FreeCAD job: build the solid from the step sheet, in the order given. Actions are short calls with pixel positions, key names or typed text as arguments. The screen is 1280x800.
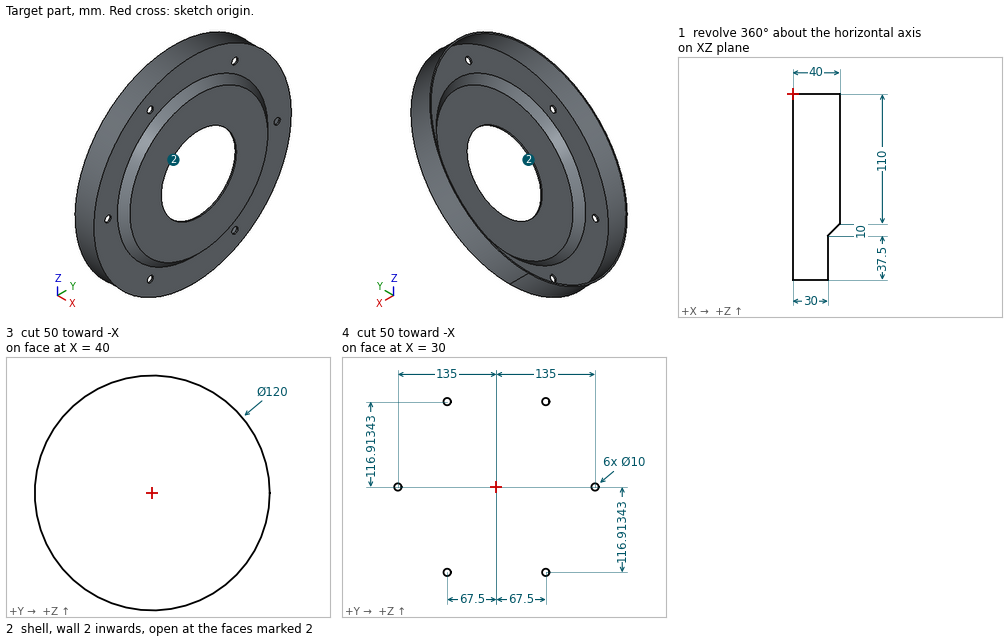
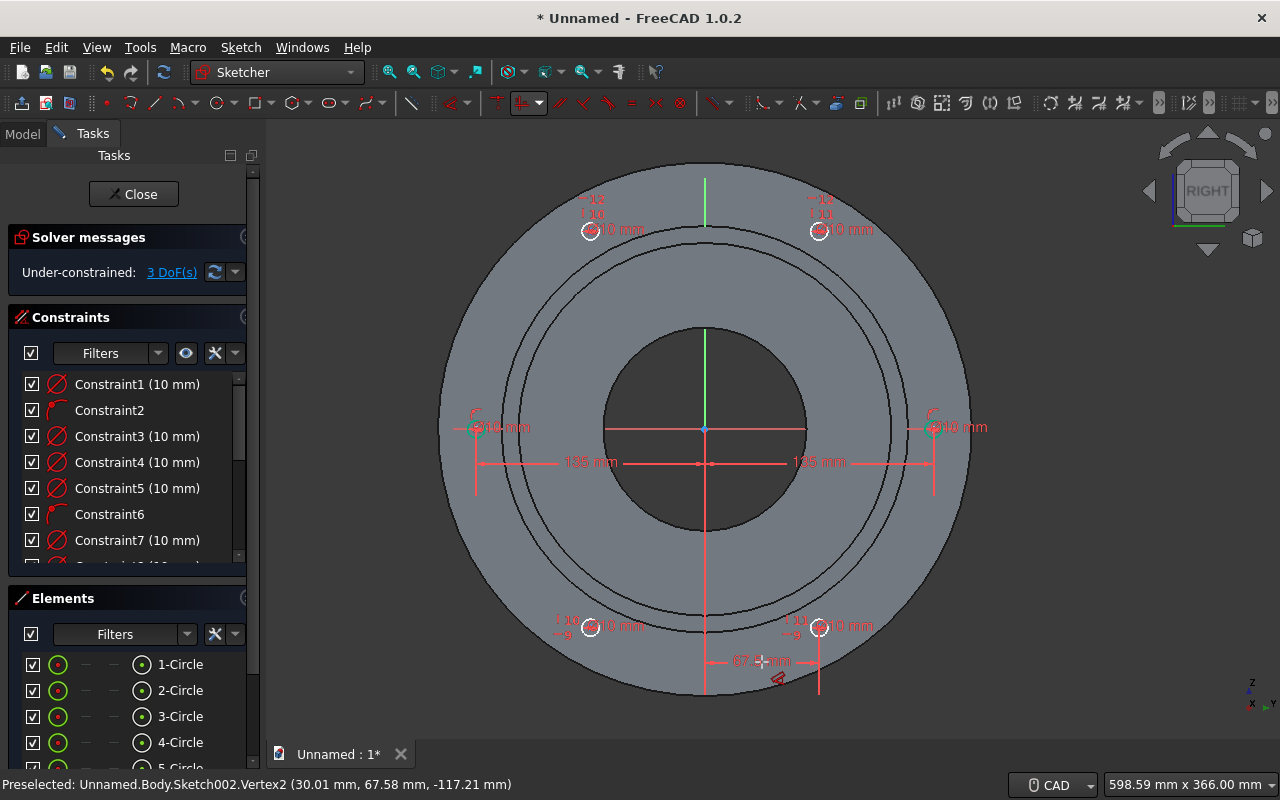
click(590, 628)
click(648, 662)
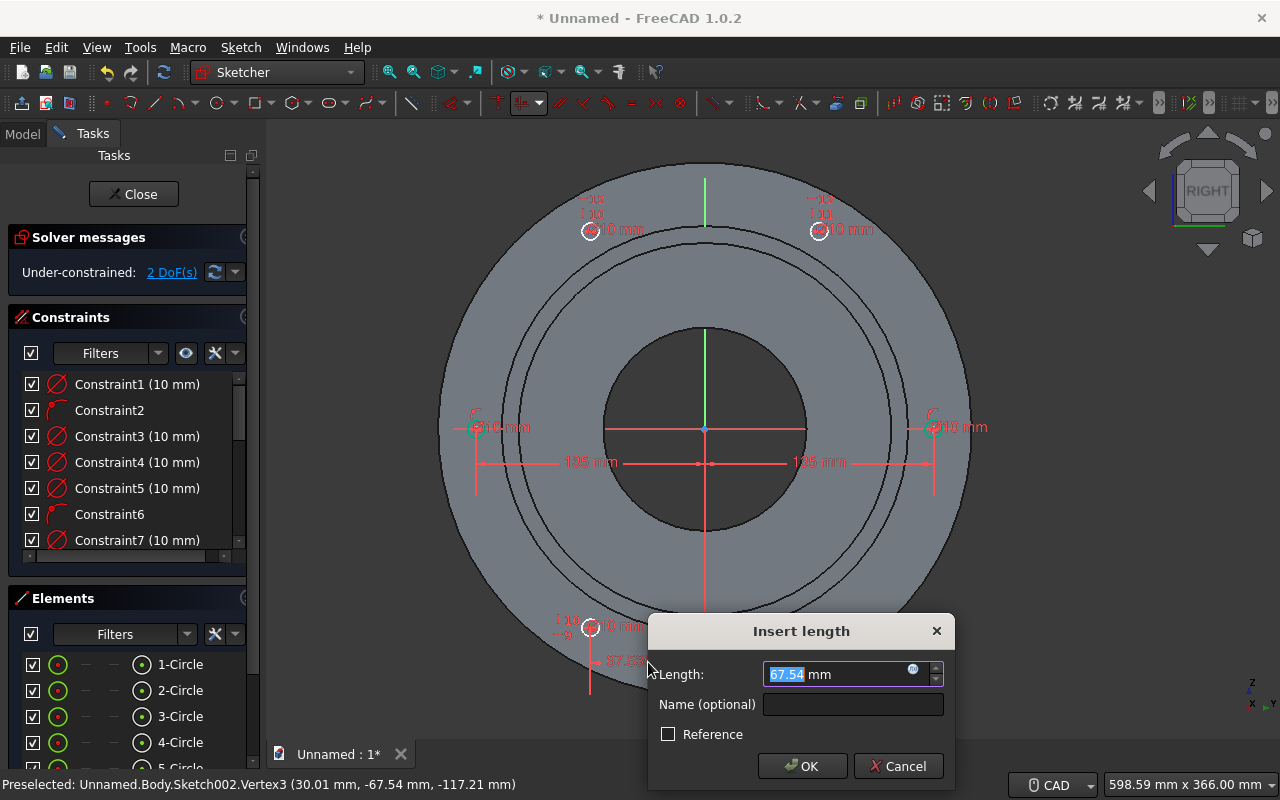
text(67.5)
key(Return)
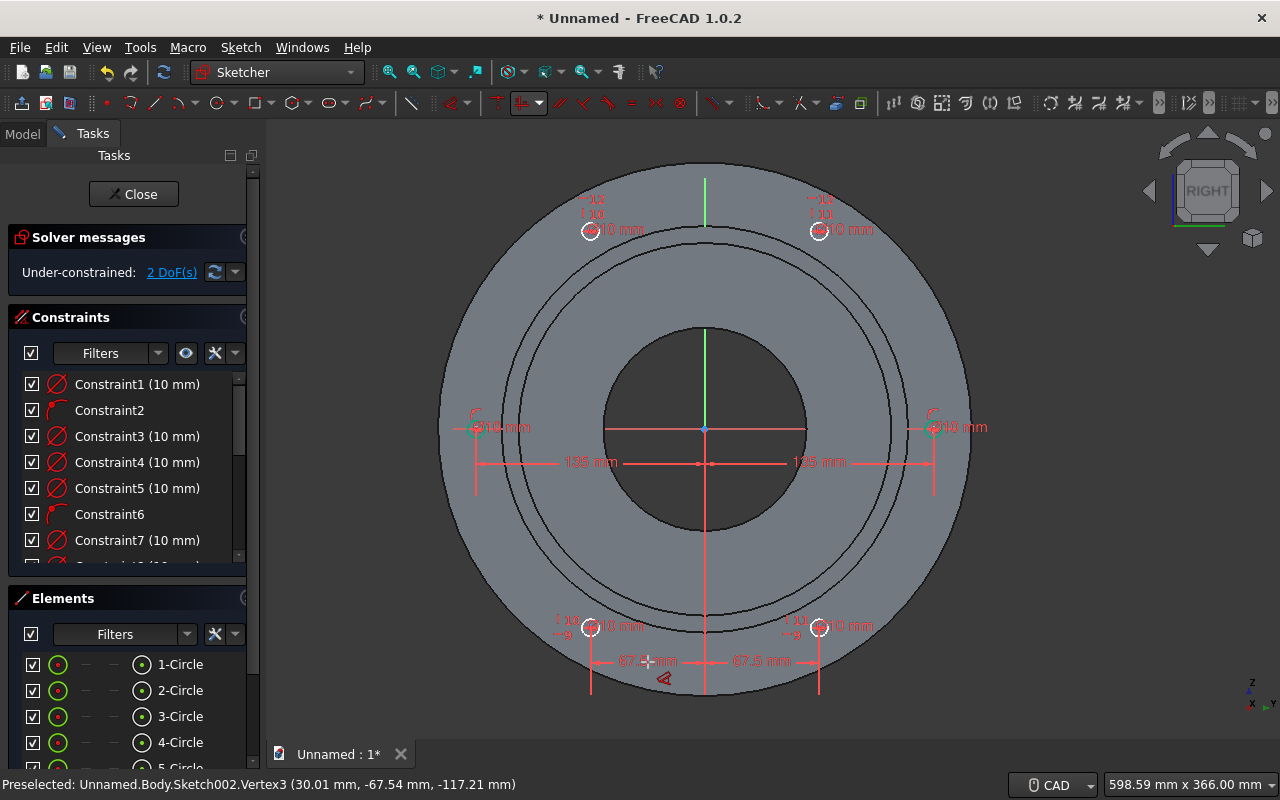
click(819, 628)
click(853, 529)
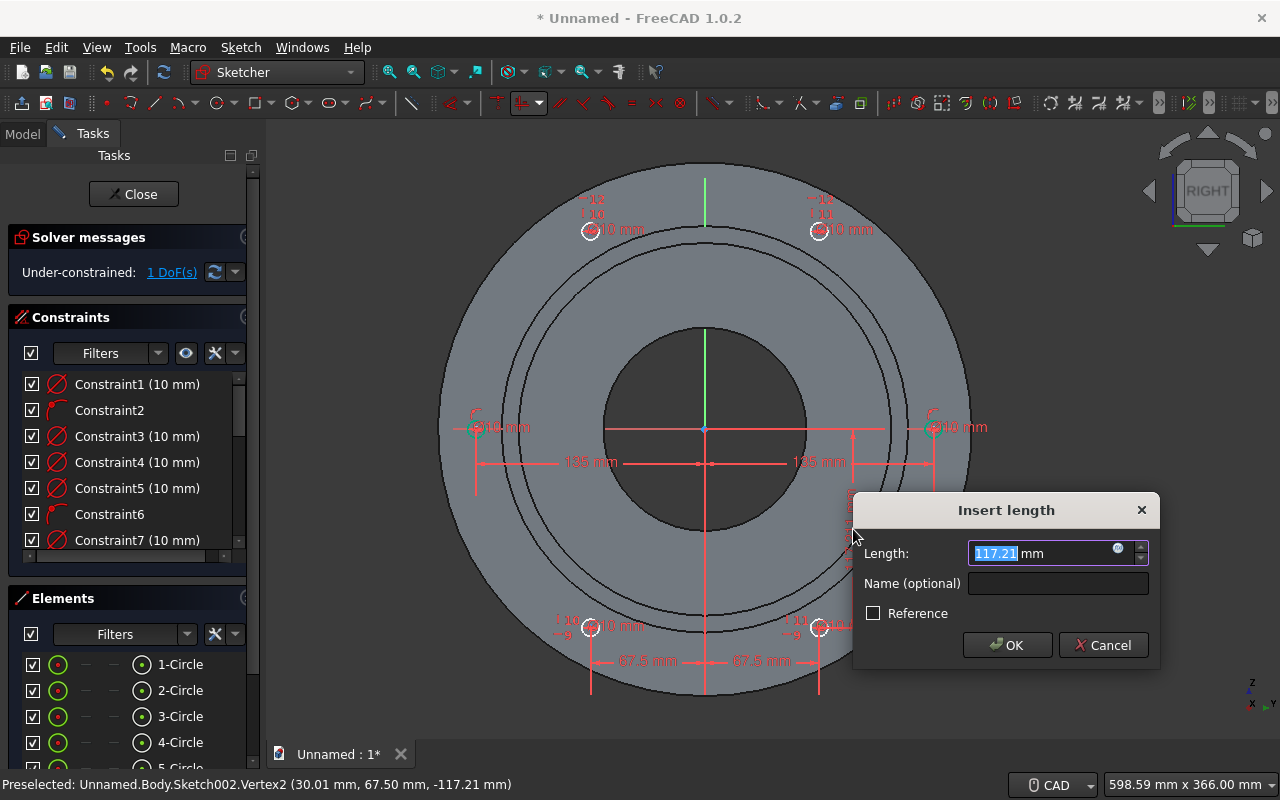
text(116.91343)
key(Return)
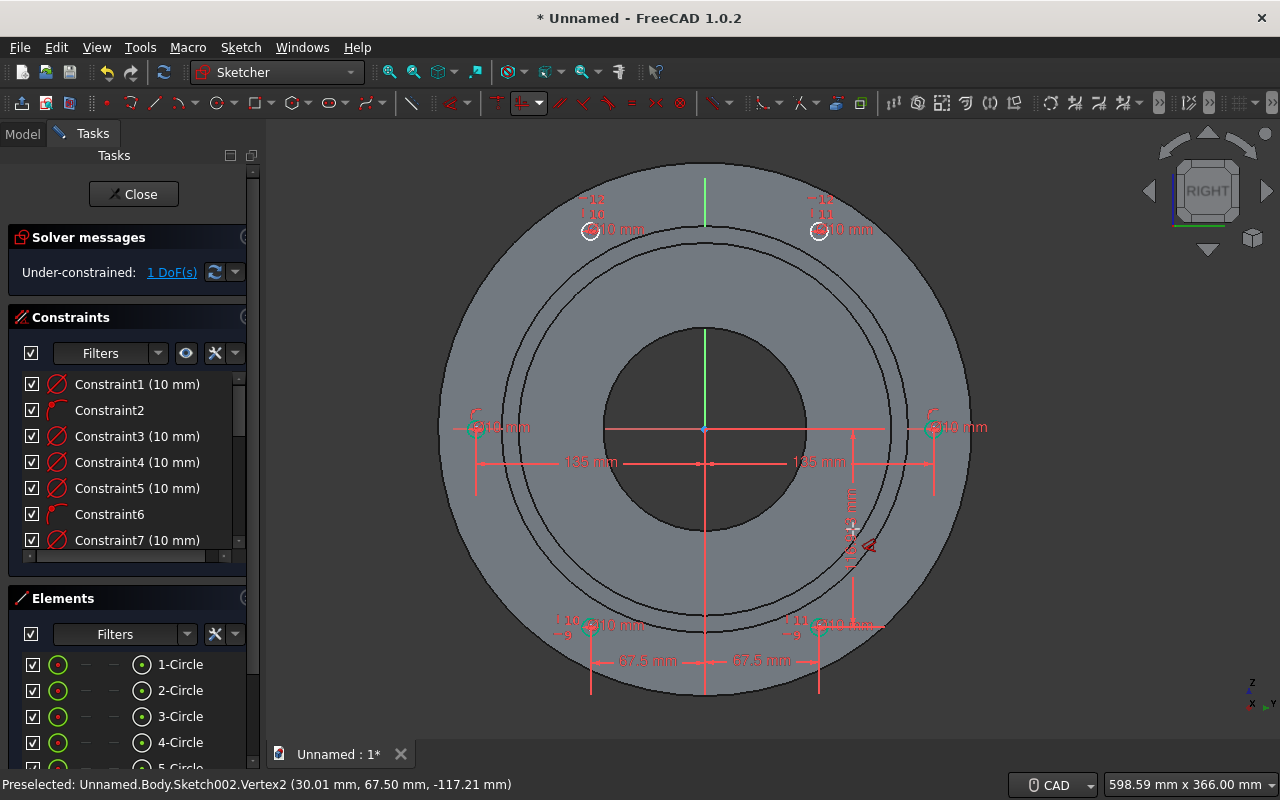
click(591, 231)
click(557, 330)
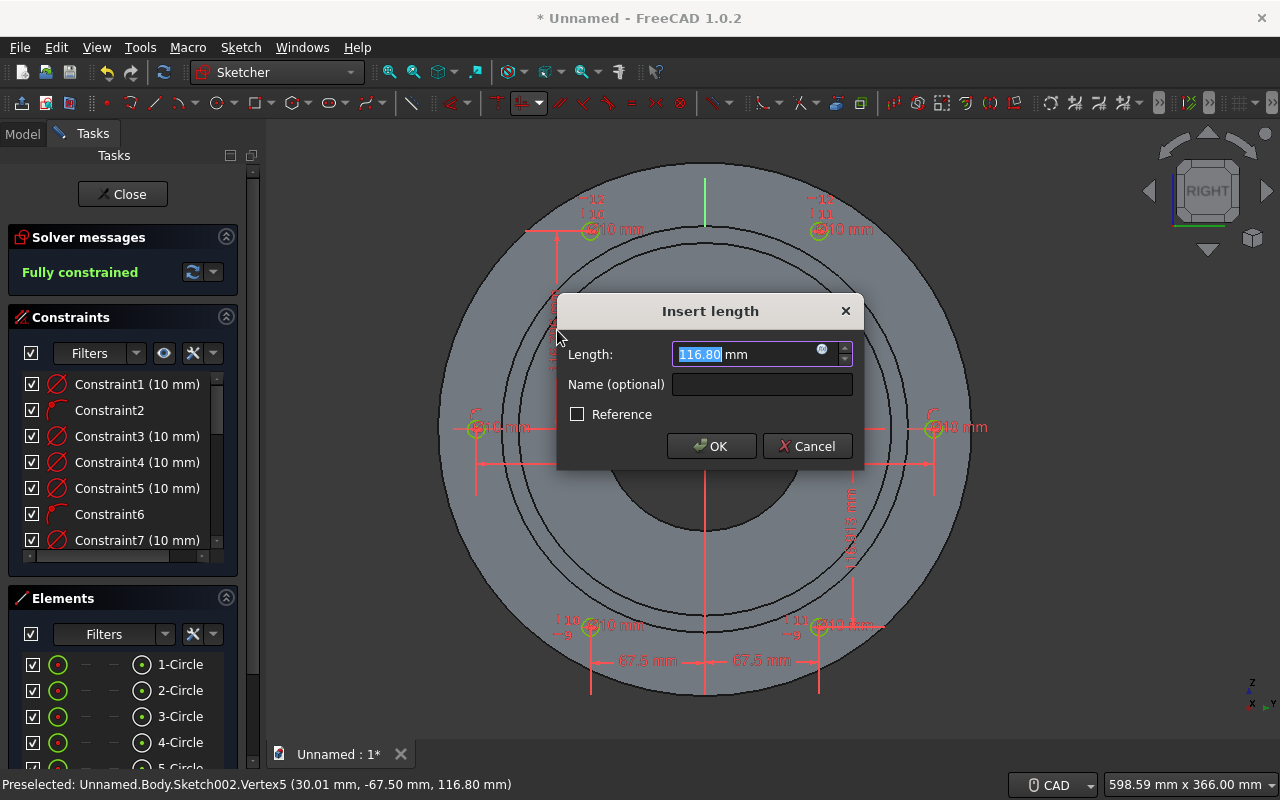
text(116.91343)
key(Return)
key(Escape)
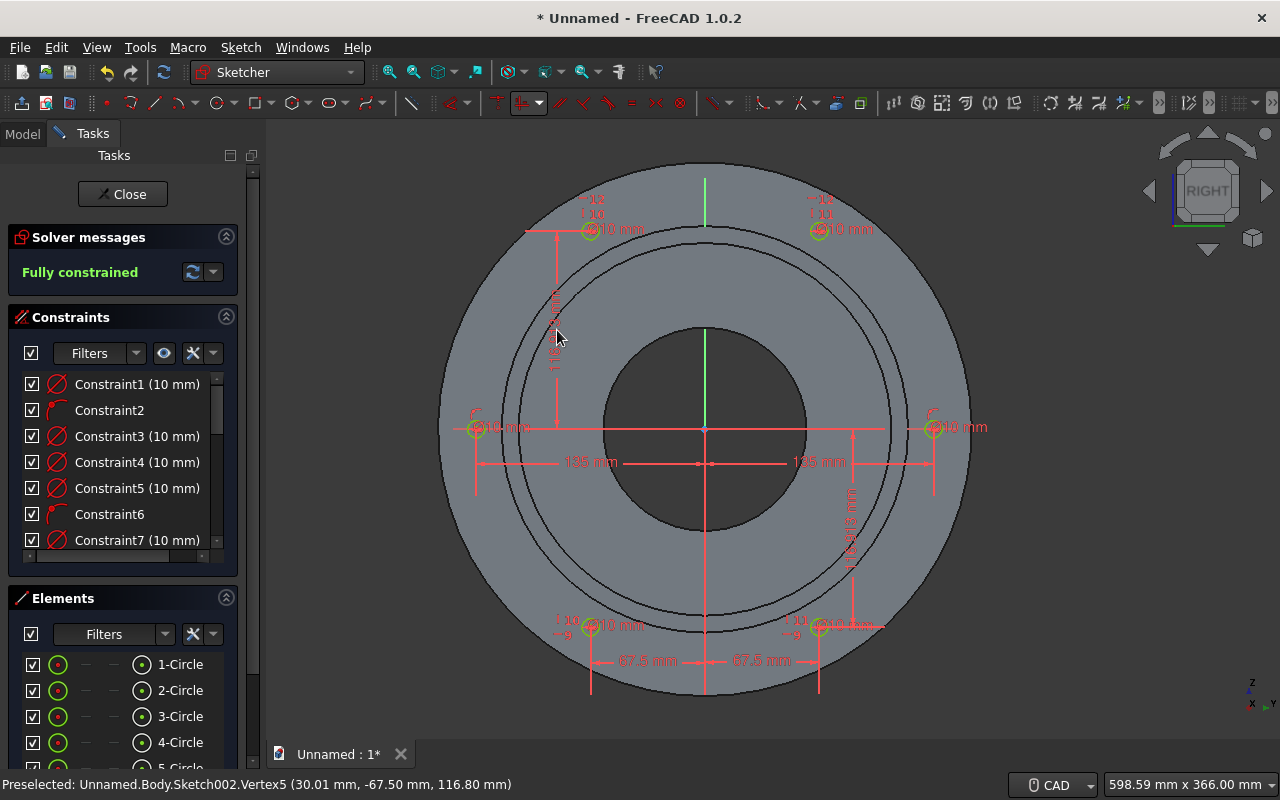
click(123, 194)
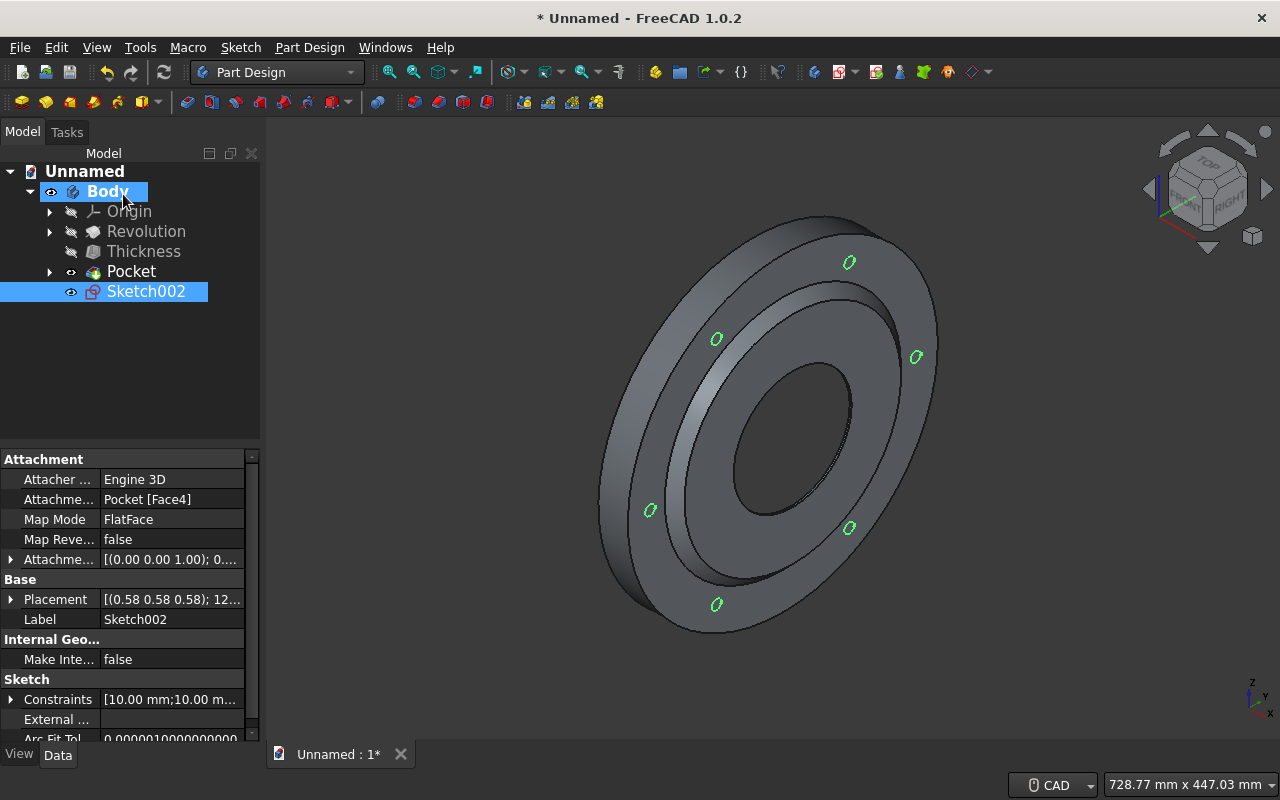
click(188, 102)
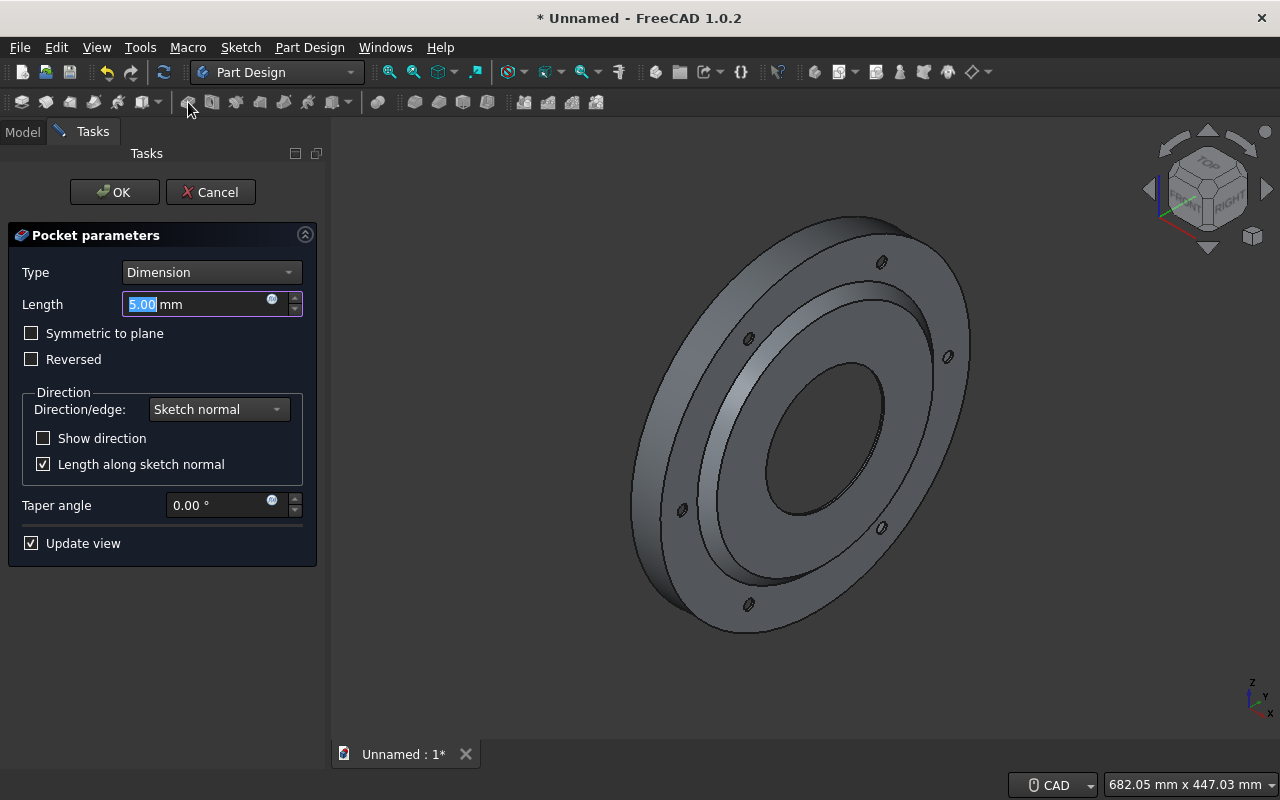
text(50)
key(Tab)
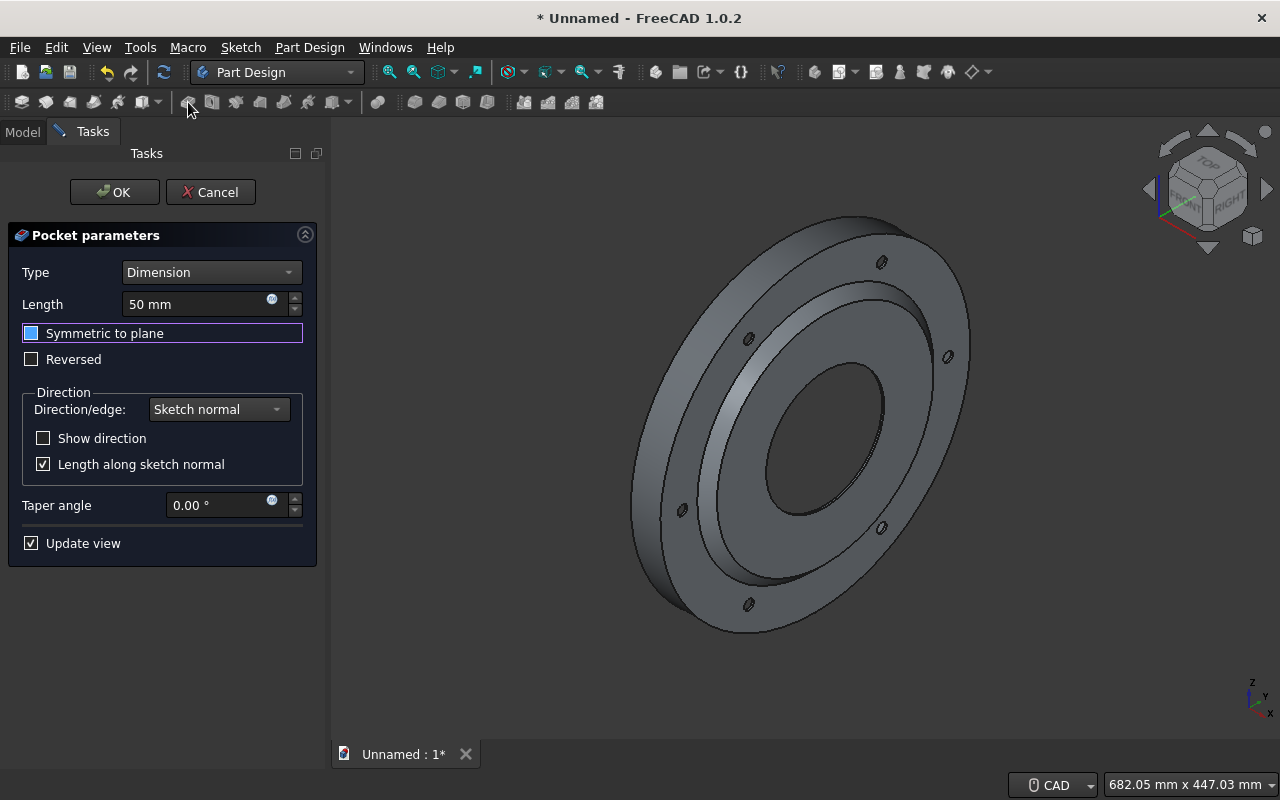
click(115, 192)